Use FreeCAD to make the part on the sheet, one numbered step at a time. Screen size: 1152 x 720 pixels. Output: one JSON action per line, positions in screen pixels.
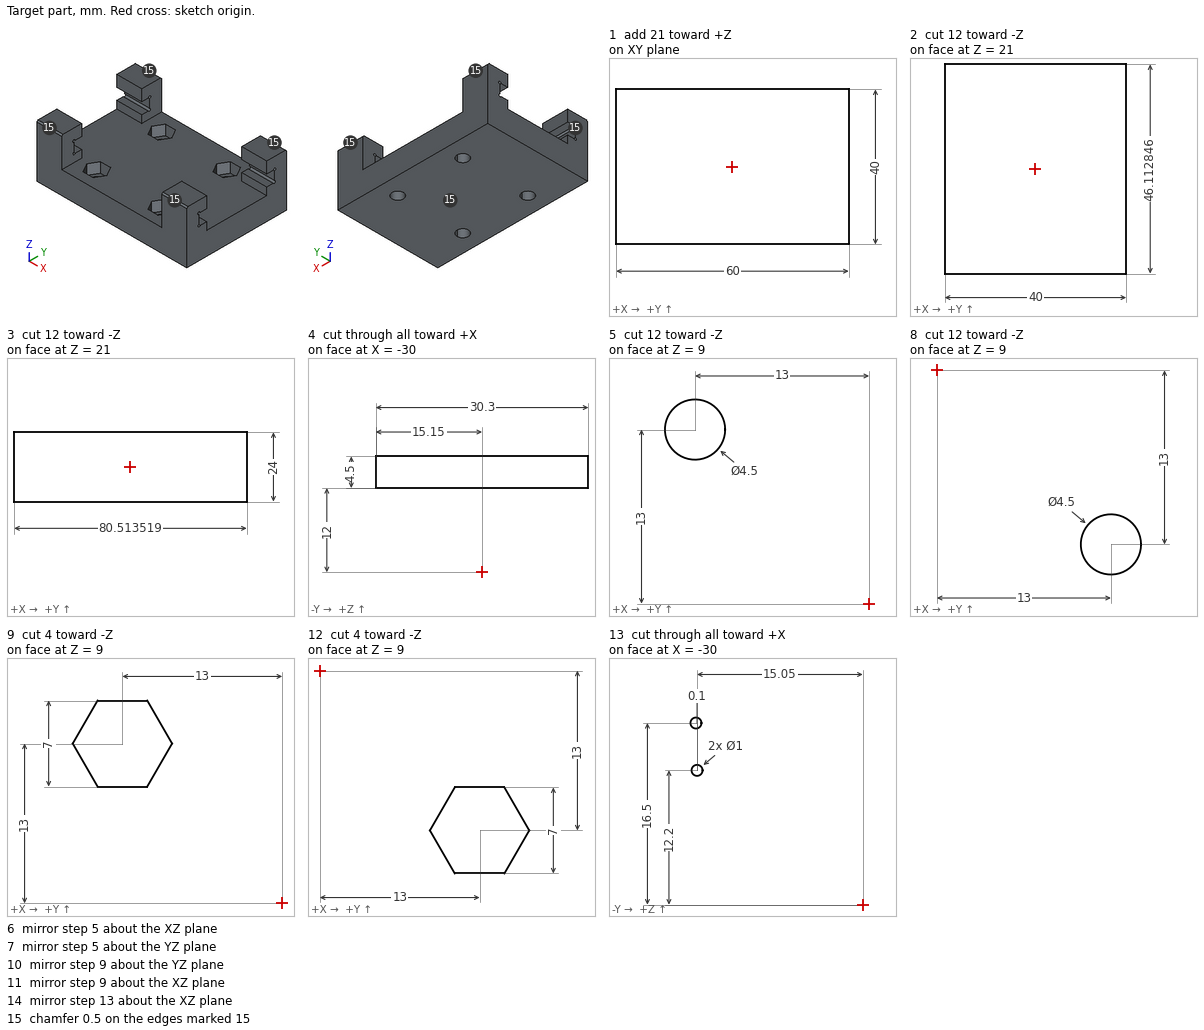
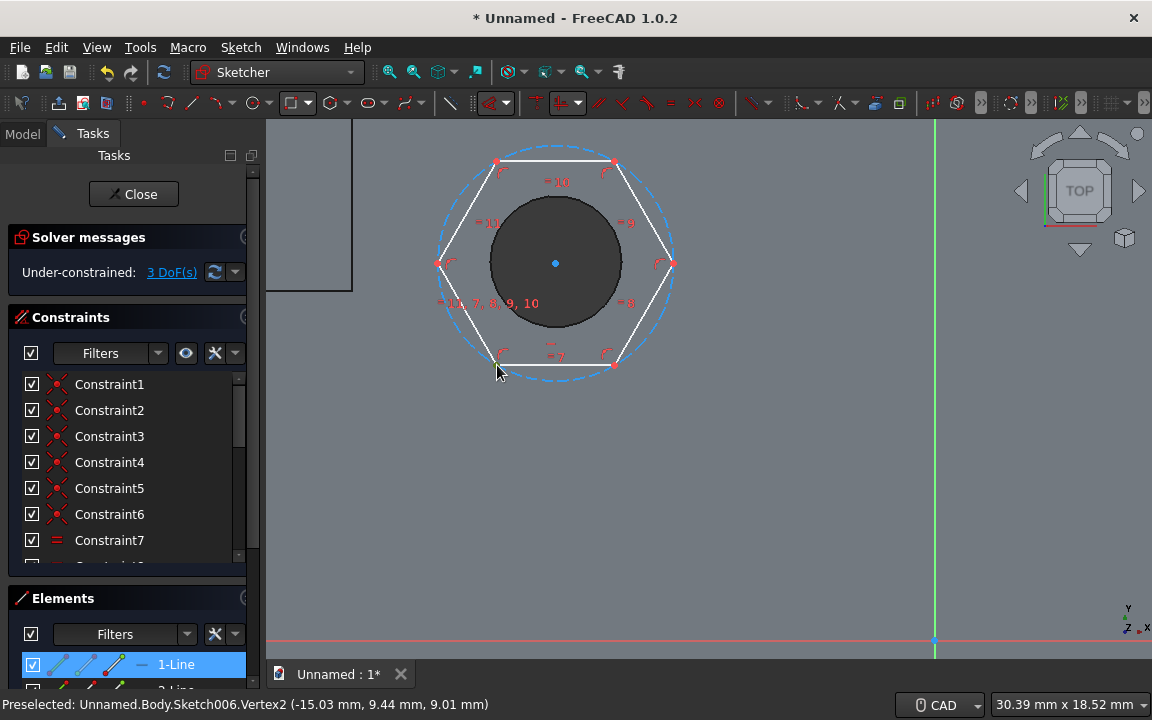
{"action": "left_click", "coordinate": [615, 161]}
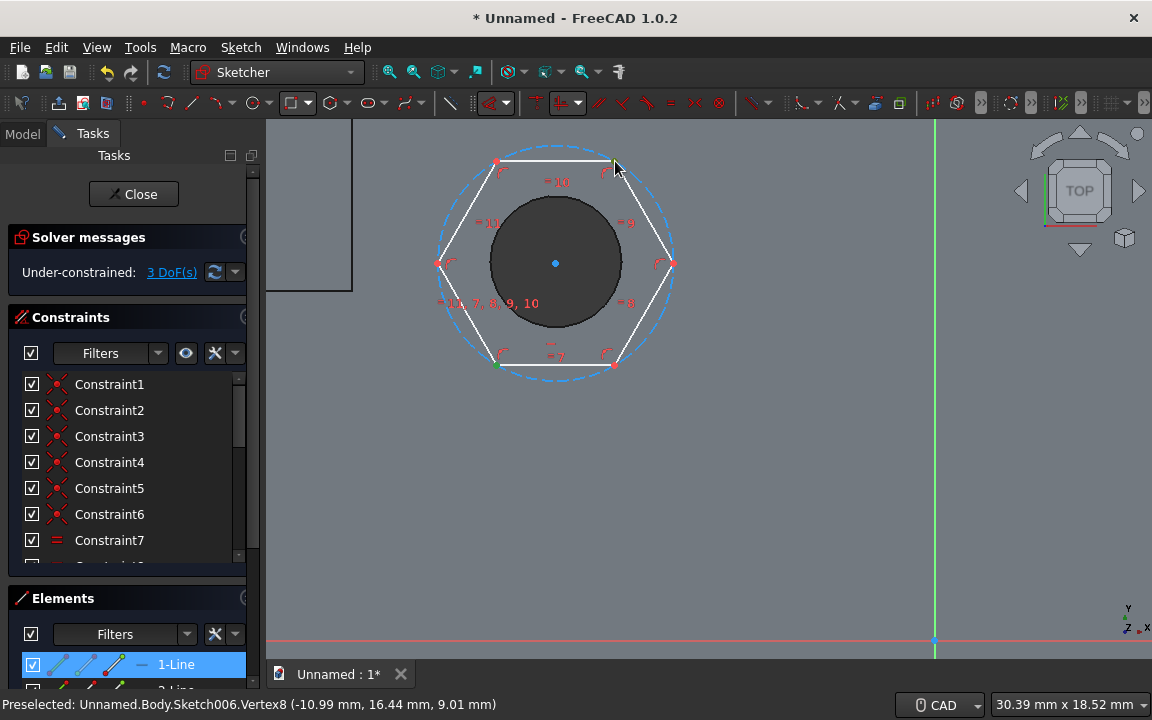
{"action": "left_click", "coordinate": [508, 104]}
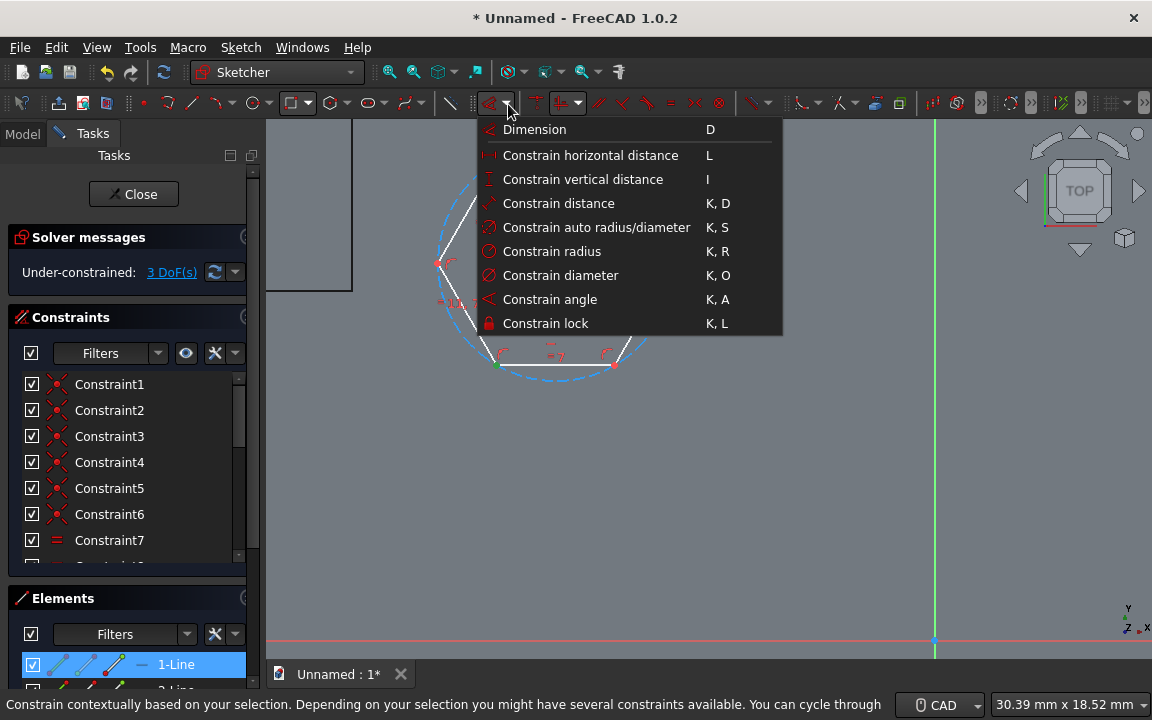
{"action": "left_click", "coordinate": [630, 179]}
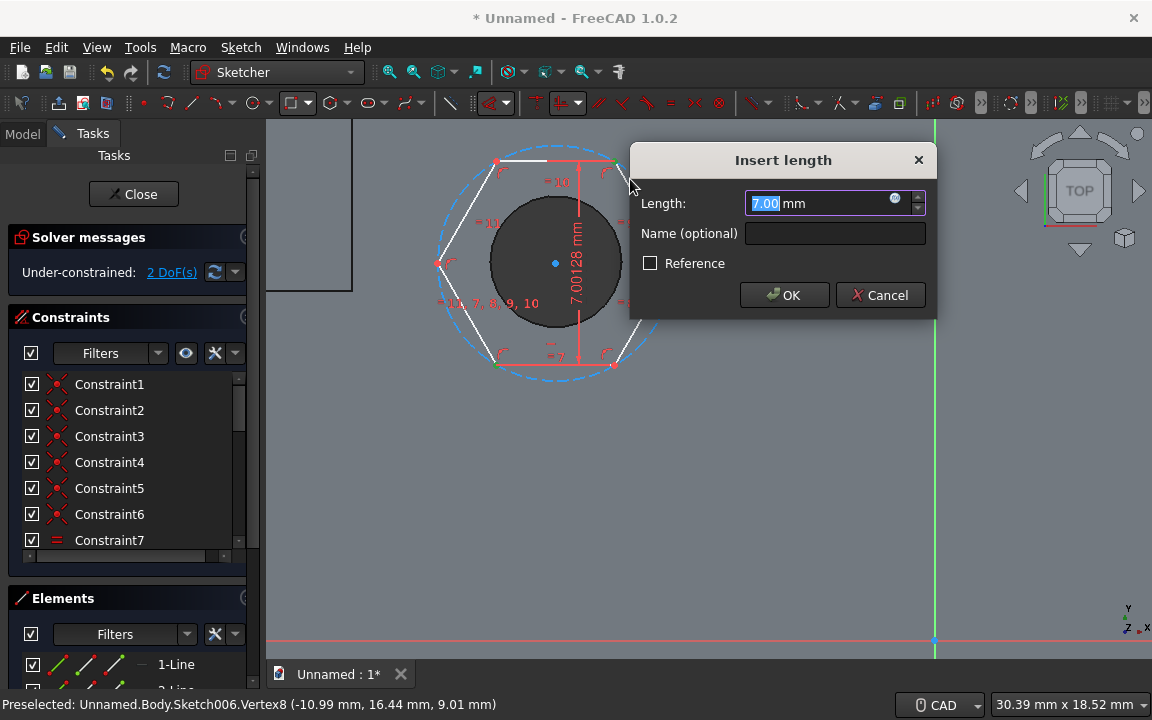
{"action": "type", "text": "7"}
{"action": "key", "text": "Return"}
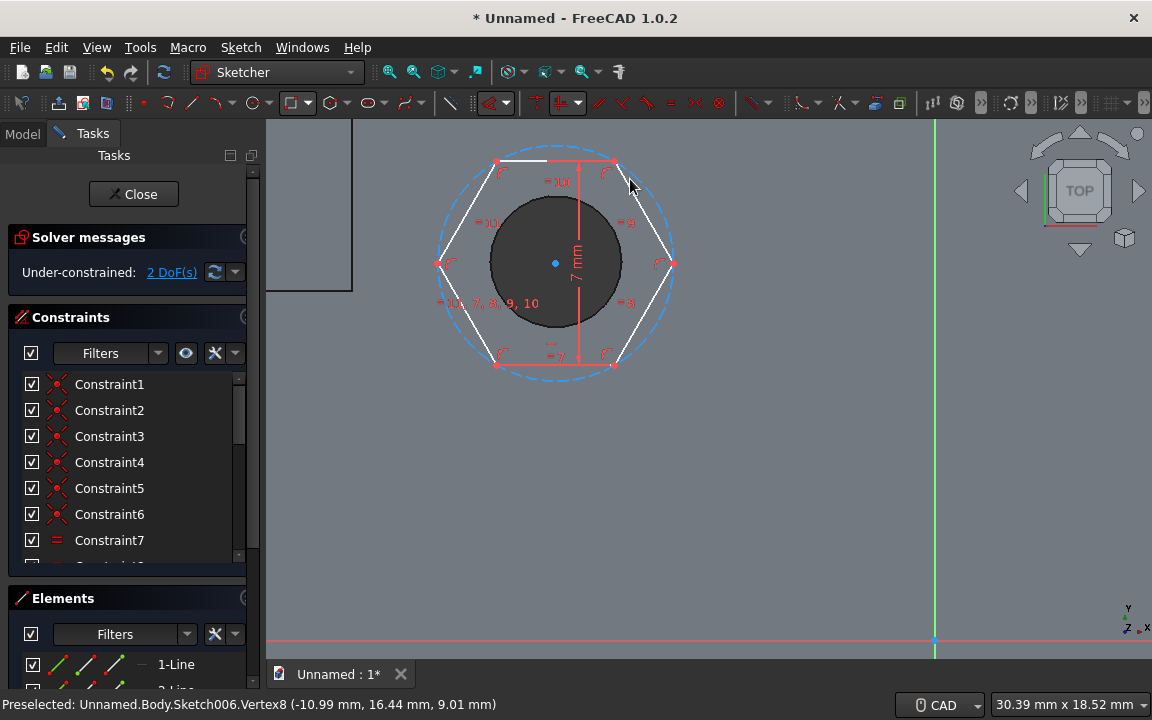
{"action": "left_click", "coordinate": [556, 263]}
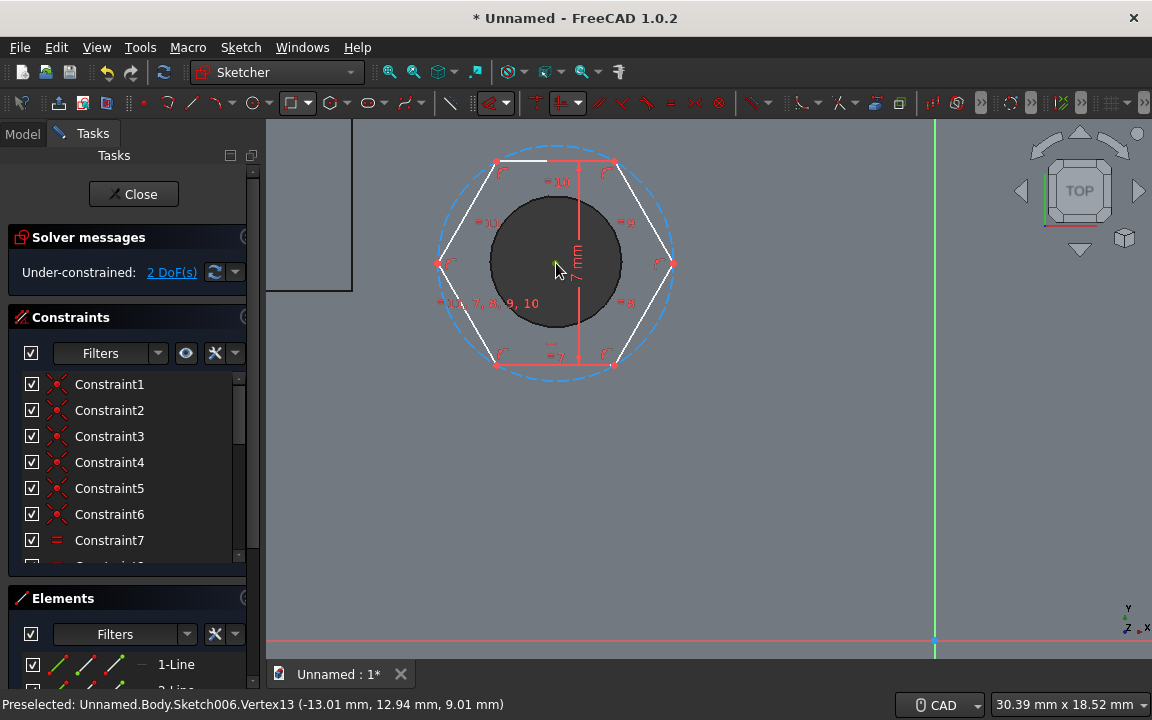
{"action": "key", "text": "l"}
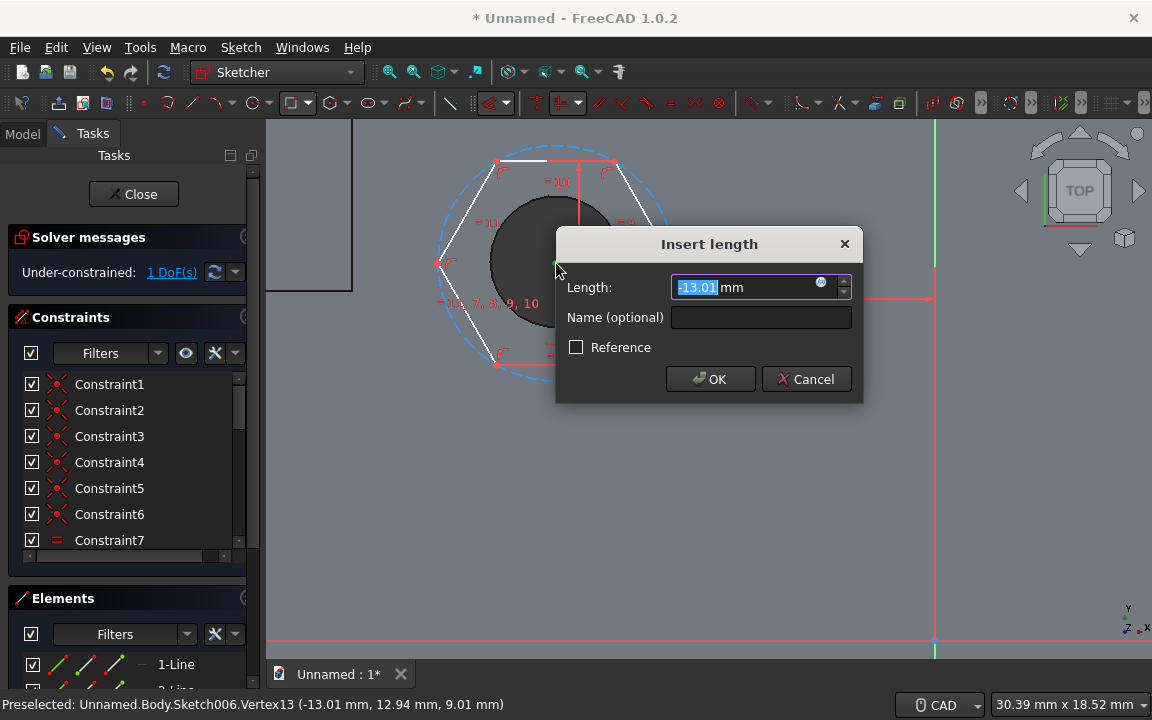
{"action": "type", "text": "-13"}
{"action": "key", "text": "Return"}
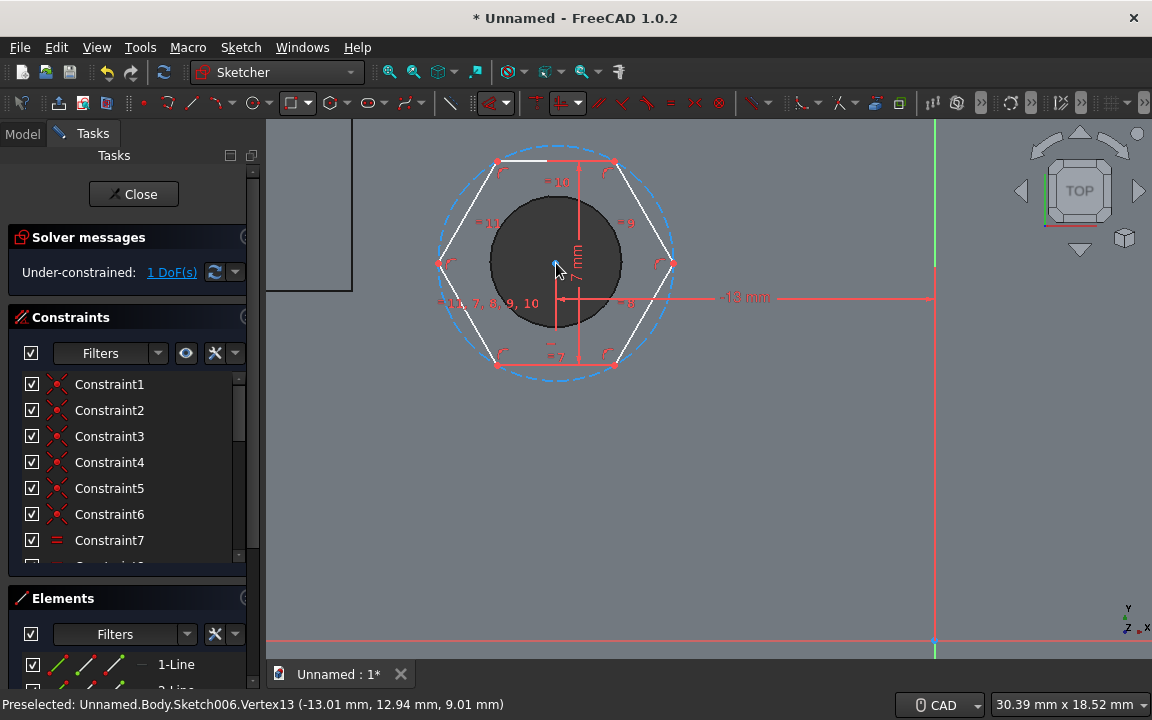
{"action": "left_click", "coordinate": [556, 263]}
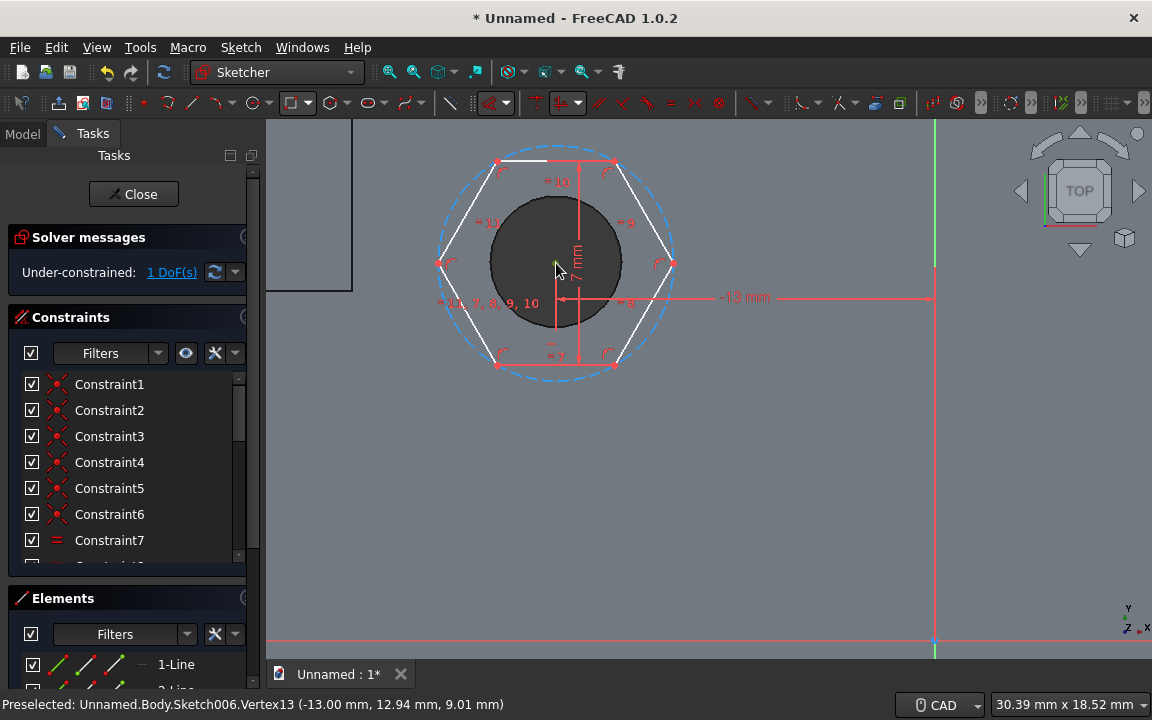
{"action": "left_click", "coordinate": [508, 104]}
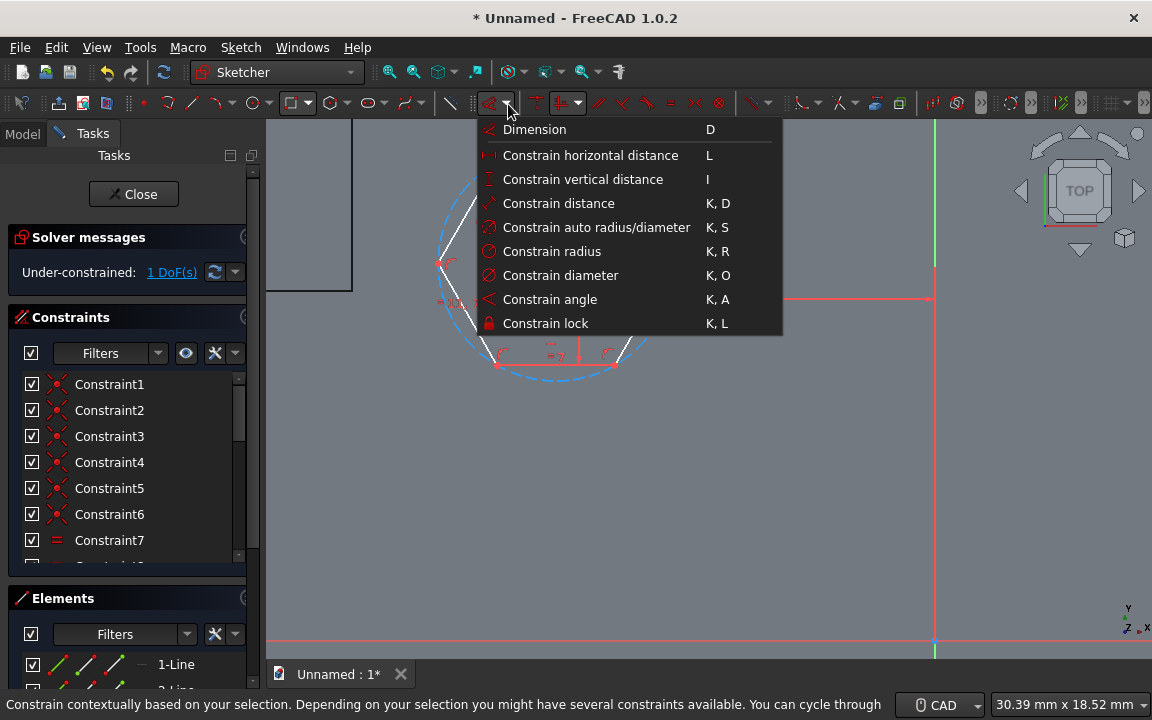
{"action": "left_click", "coordinate": [630, 179]}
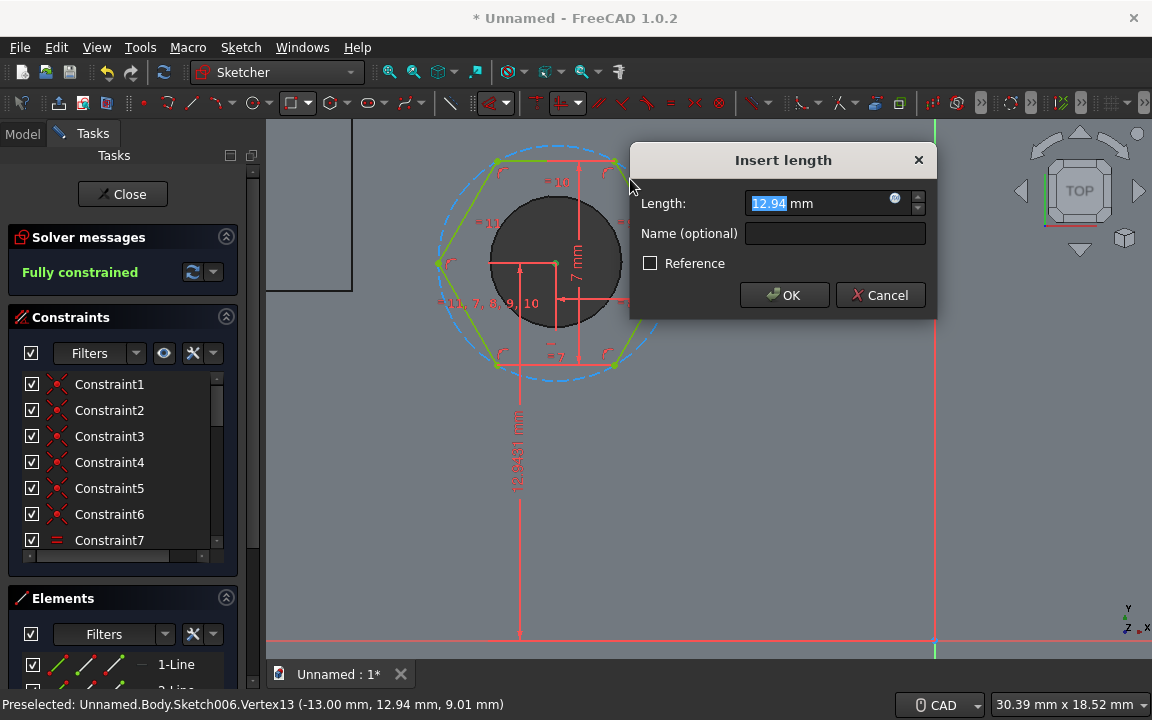
{"action": "type", "text": "13"}
{"action": "key", "text": "Return"}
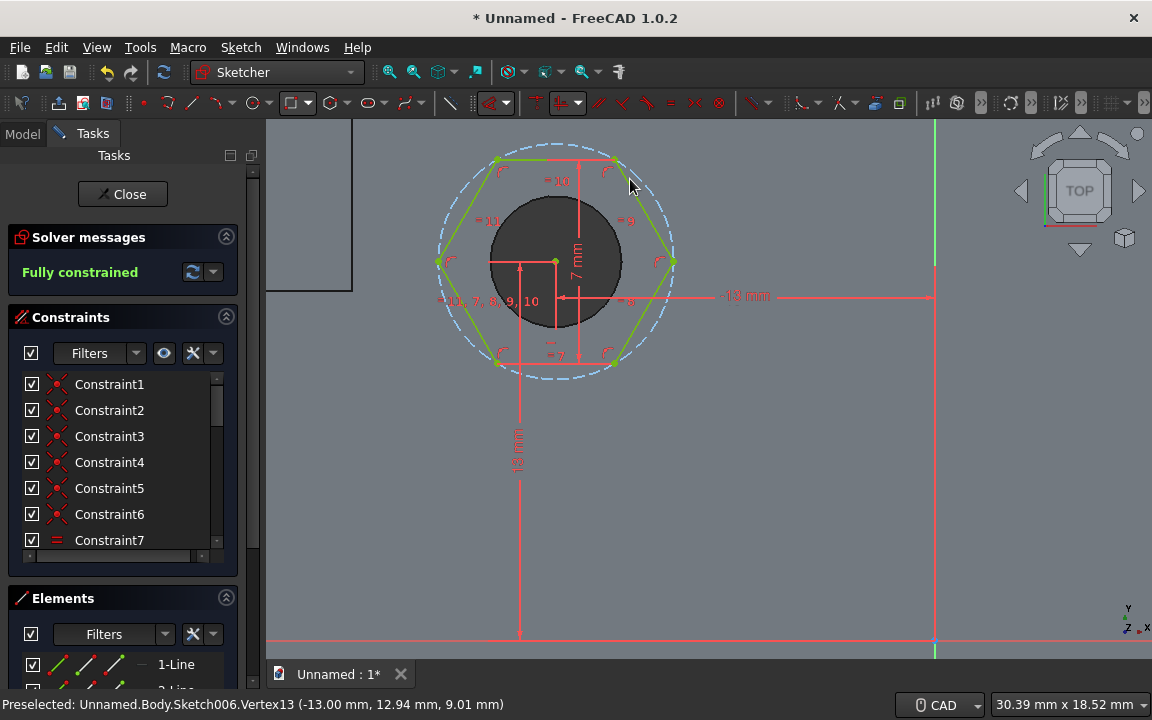
{"action": "left_click", "coordinate": [123, 194]}